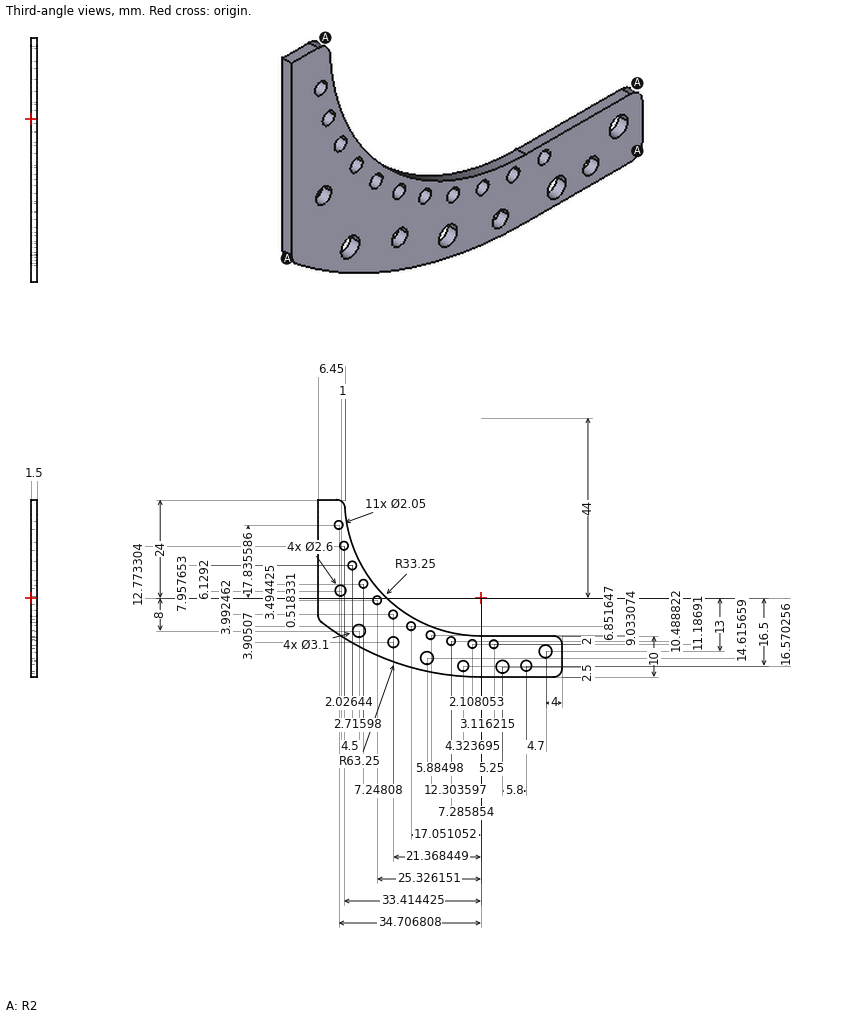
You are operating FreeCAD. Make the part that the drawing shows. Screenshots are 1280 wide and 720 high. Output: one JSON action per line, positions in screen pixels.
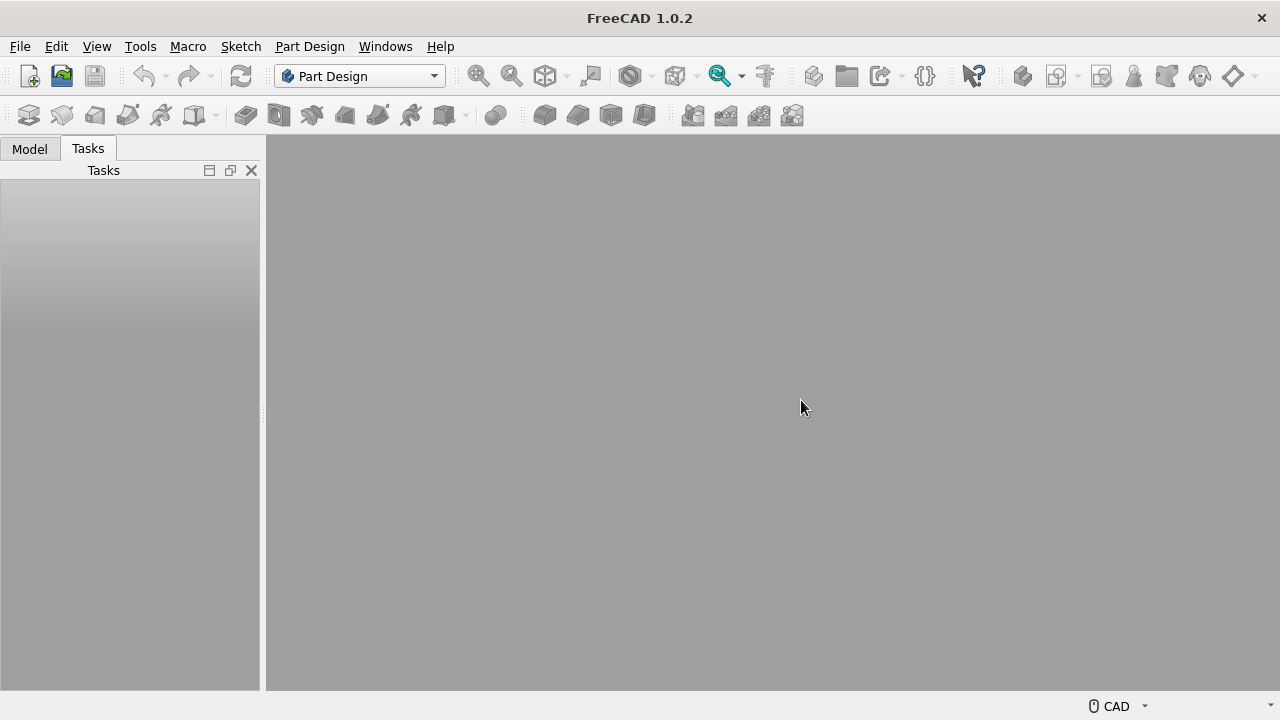
{"action": "left_click", "coordinate": [29, 76]}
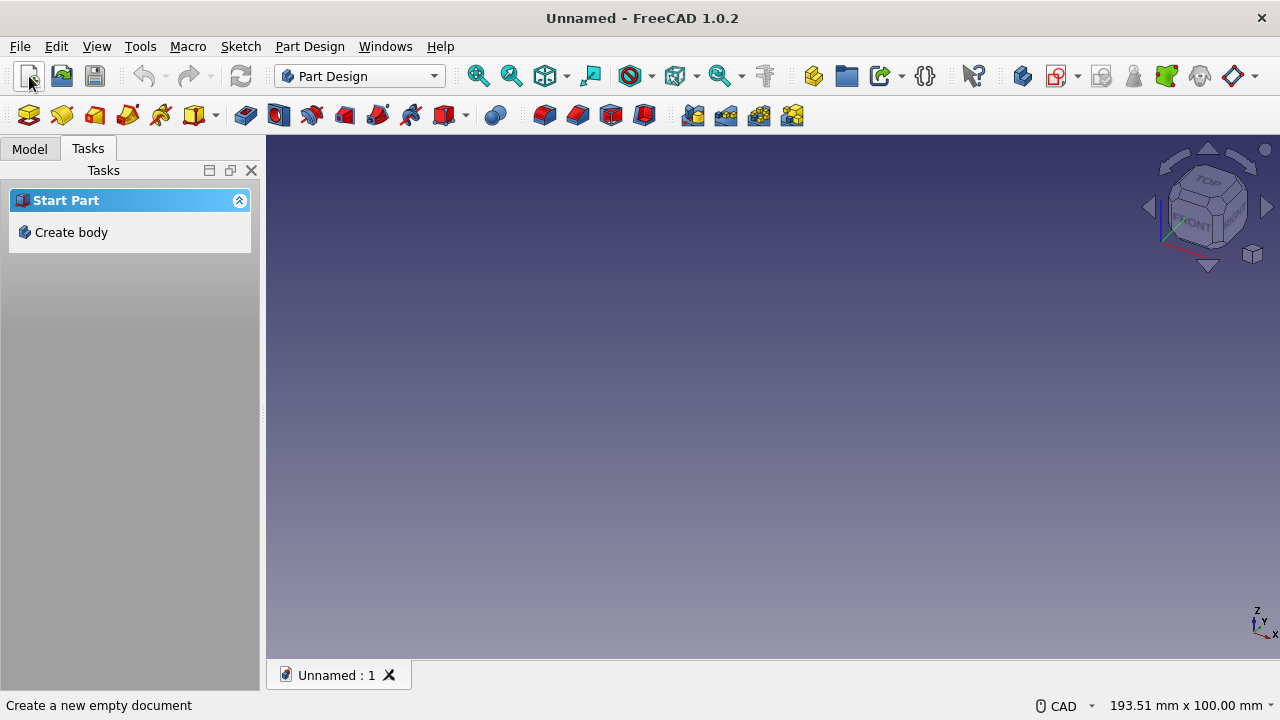
{"action": "left_click", "coordinate": [1056, 76]}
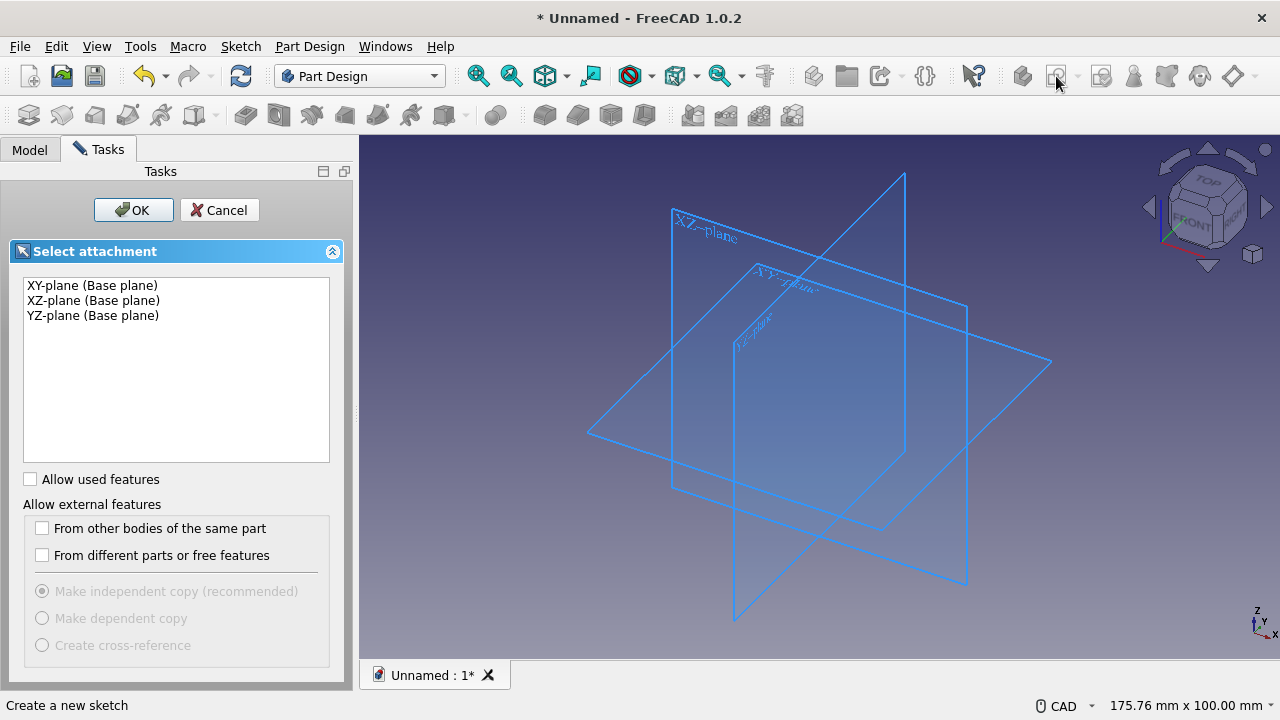
{"action": "left_click", "coordinate": [84, 316]}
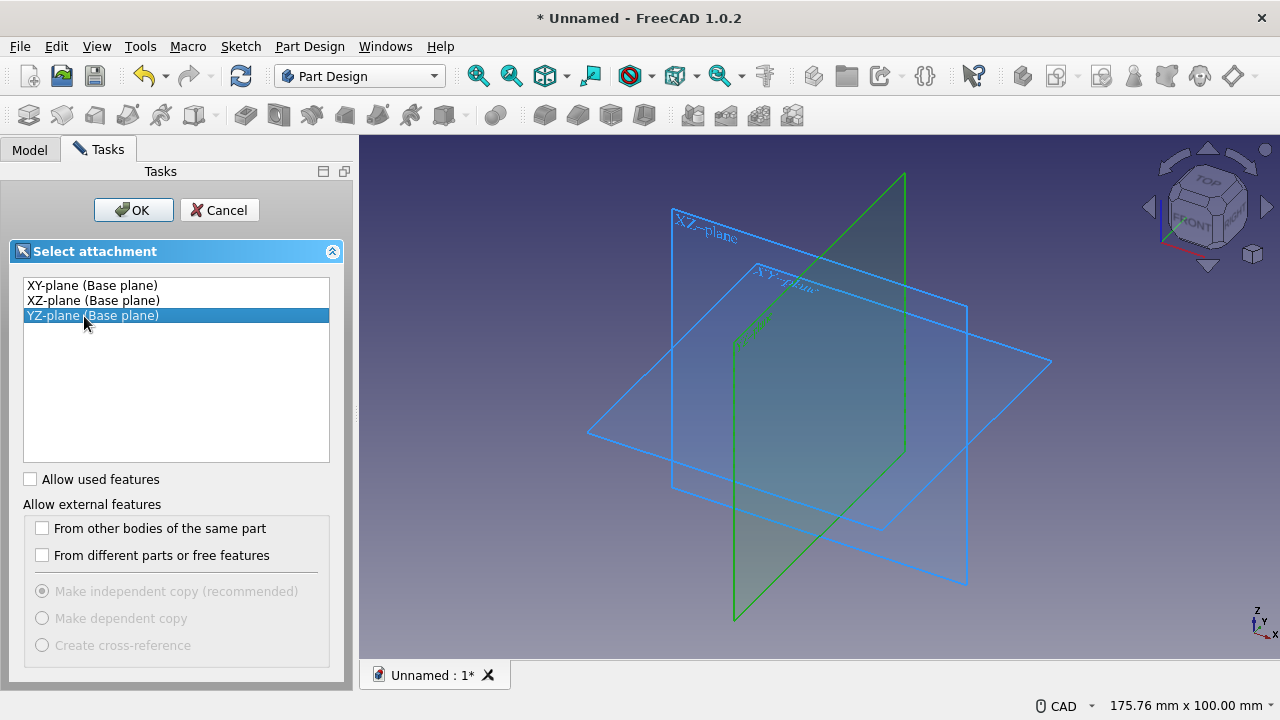
{"action": "left_click", "coordinate": [134, 210]}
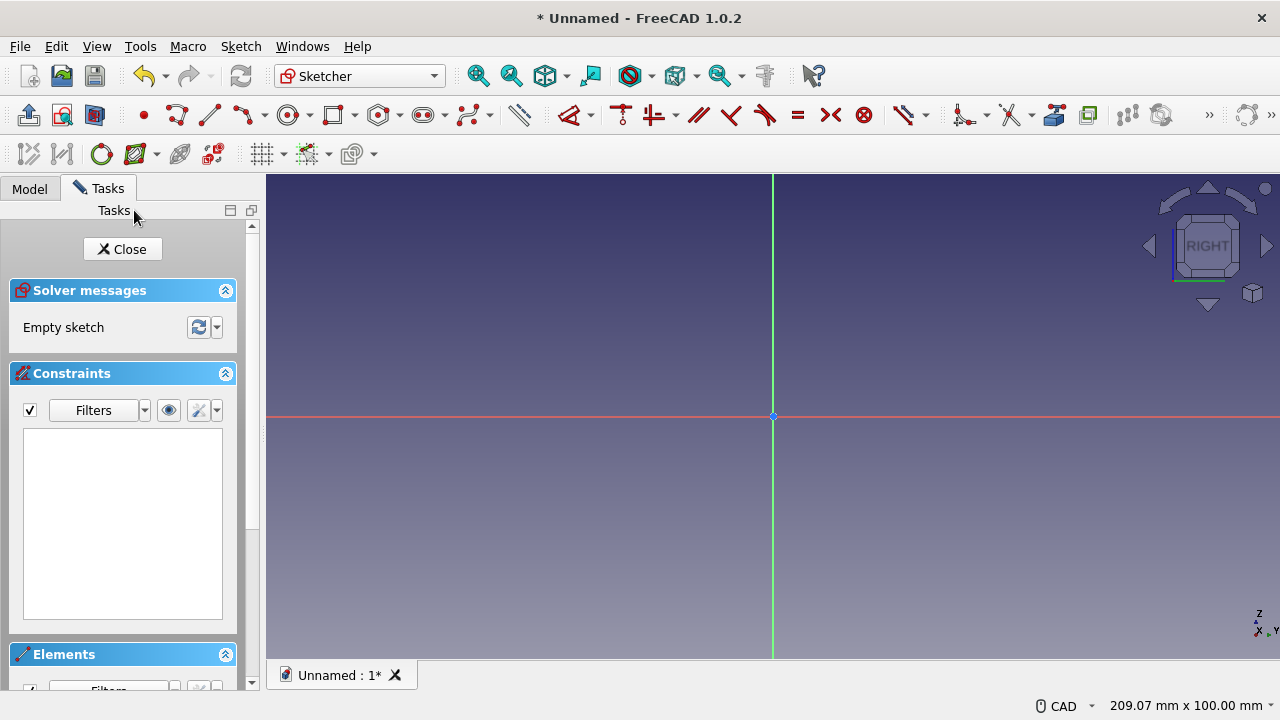
{"action": "scroll", "coordinate": [766, 382], "scroll_direction": "up", "scroll_amount": 2}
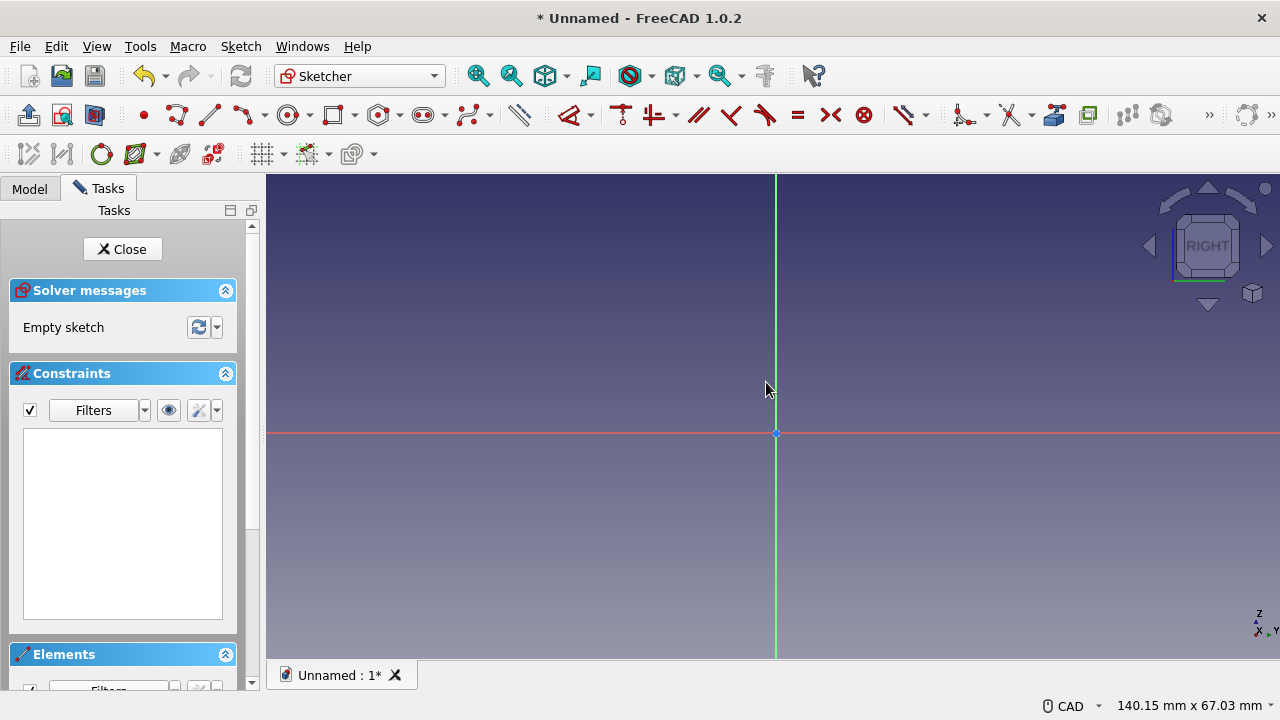
{"action": "key", "text": "g m"}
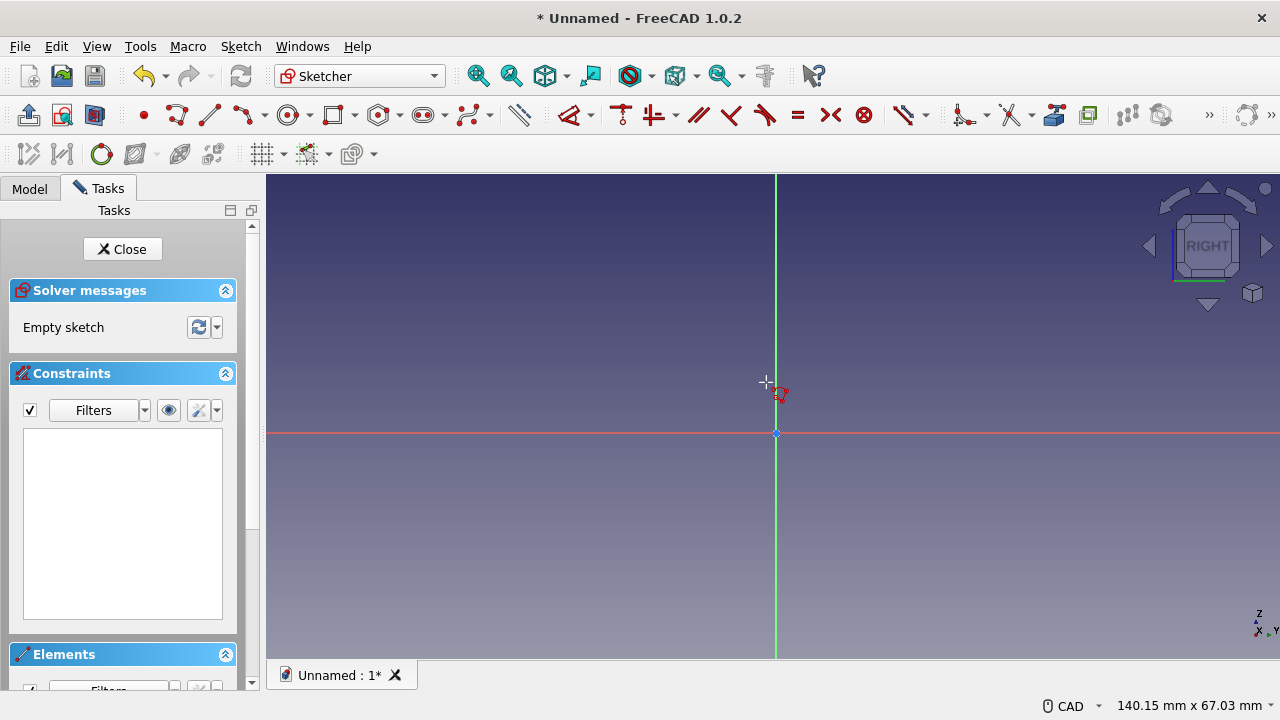
{"action": "left_click", "coordinate": [536, 260]}
{"action": "left_click", "coordinate": [489, 260]}
{"action": "left_click", "coordinate": [489, 471]}
{"action": "right_click", "coordinate": [489, 471]}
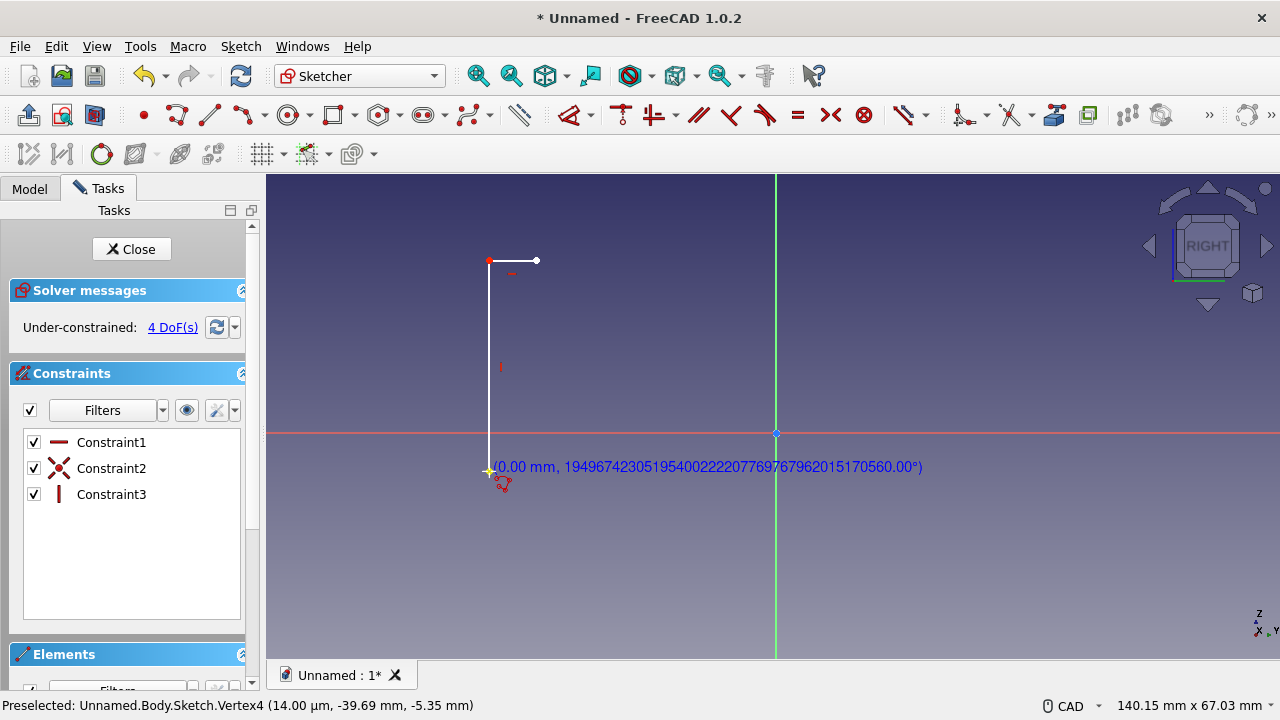
{"action": "left_click", "coordinate": [776, 573]}
{"action": "left_click", "coordinate": [919, 573]}
{"action": "left_click", "coordinate": [919, 500]}
{"action": "left_click", "coordinate": [776, 500]}
{"action": "right_click", "coordinate": [776, 500]}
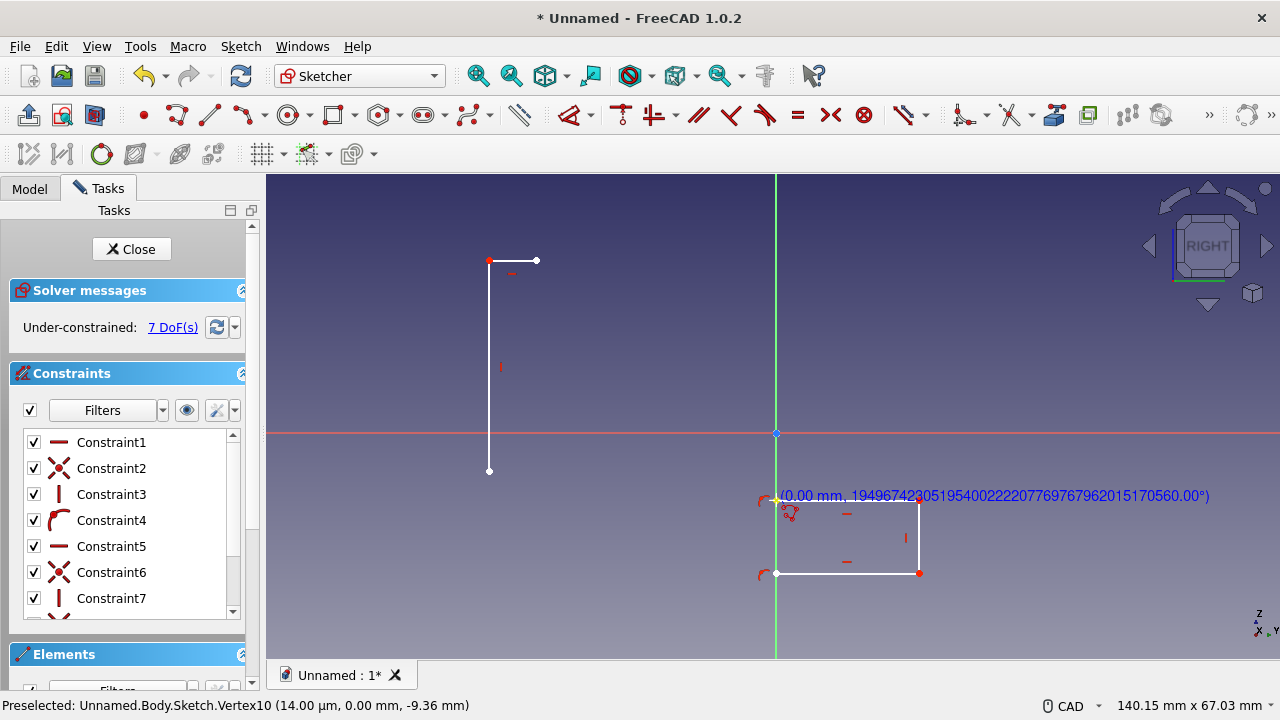
{"action": "left_click", "coordinate": [242, 116]}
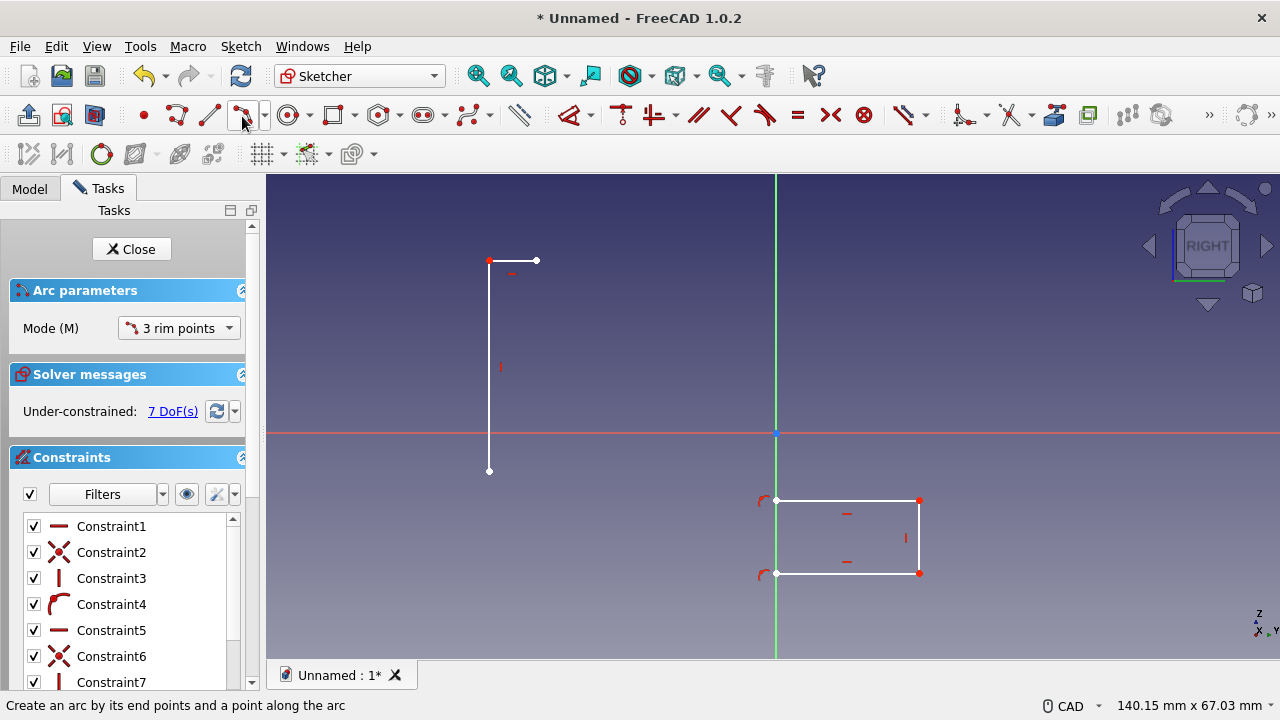
{"action": "left_click", "coordinate": [489, 472]}
{"action": "left_click", "coordinate": [776, 574]}
{"action": "left_click", "coordinate": [624, 546]}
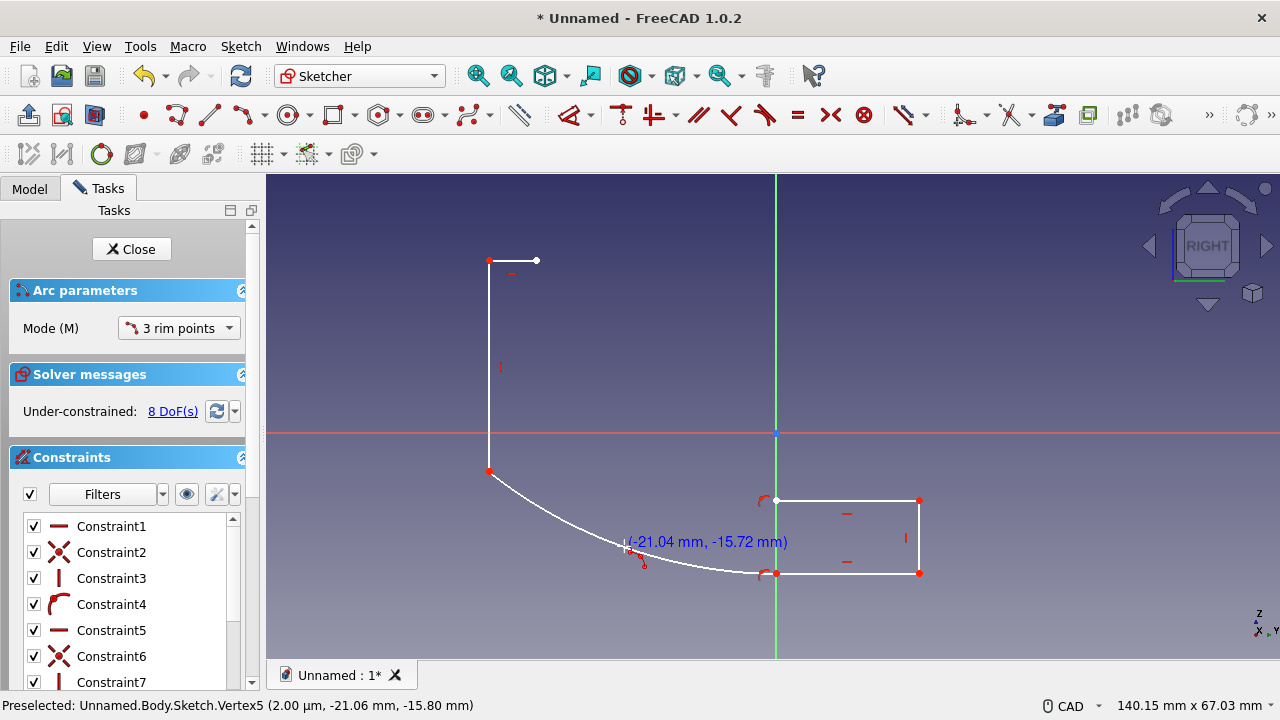
{"action": "left_click", "coordinate": [776, 501]}
{"action": "left_click", "coordinate": [536, 261]}
{"action": "left_click", "coordinate": [582, 401]}